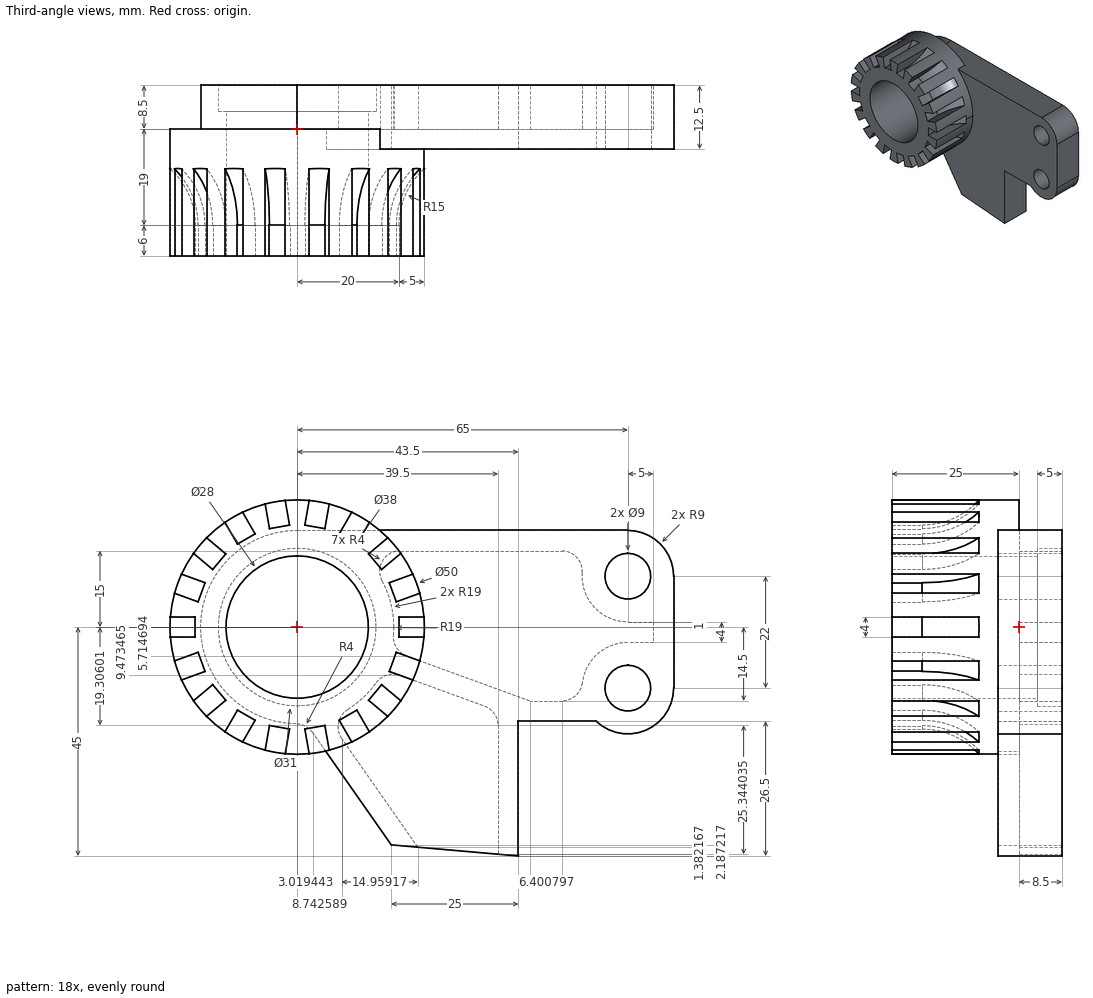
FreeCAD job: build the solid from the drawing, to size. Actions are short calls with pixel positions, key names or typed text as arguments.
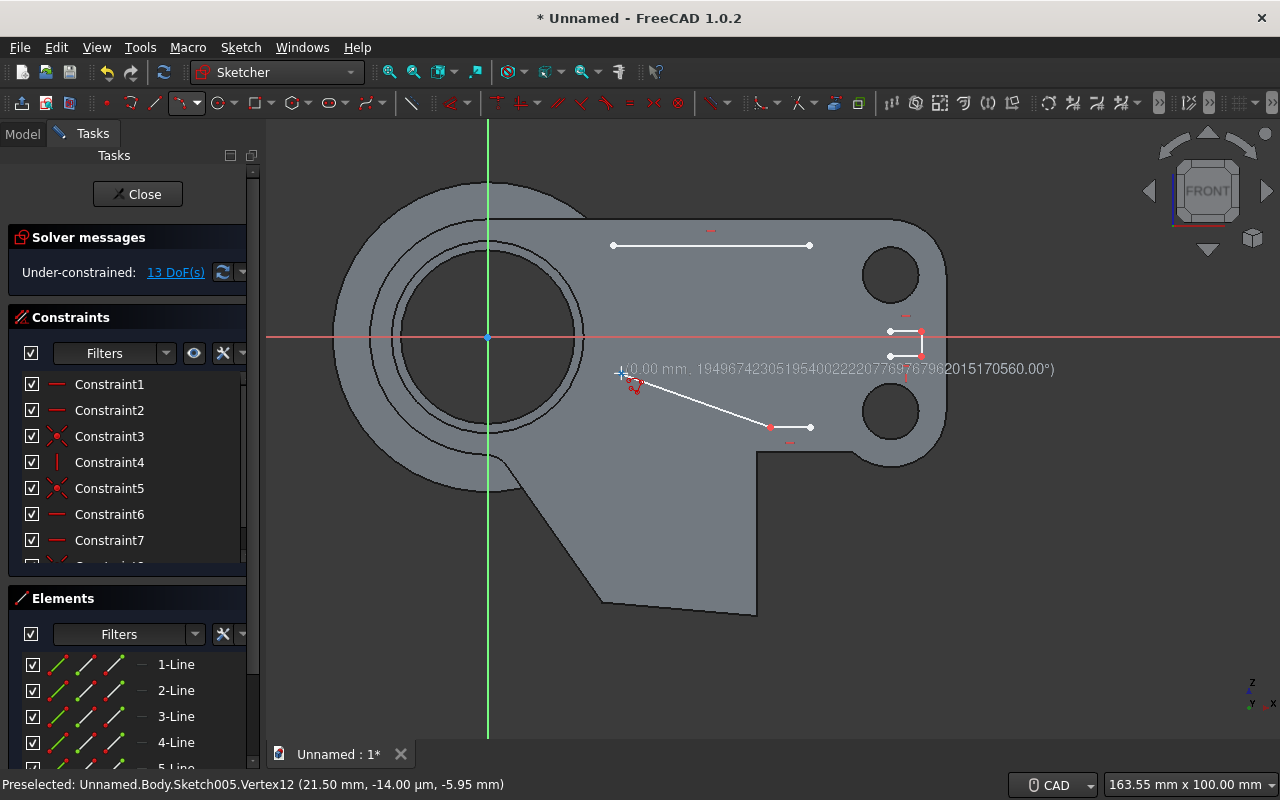
click(180, 104)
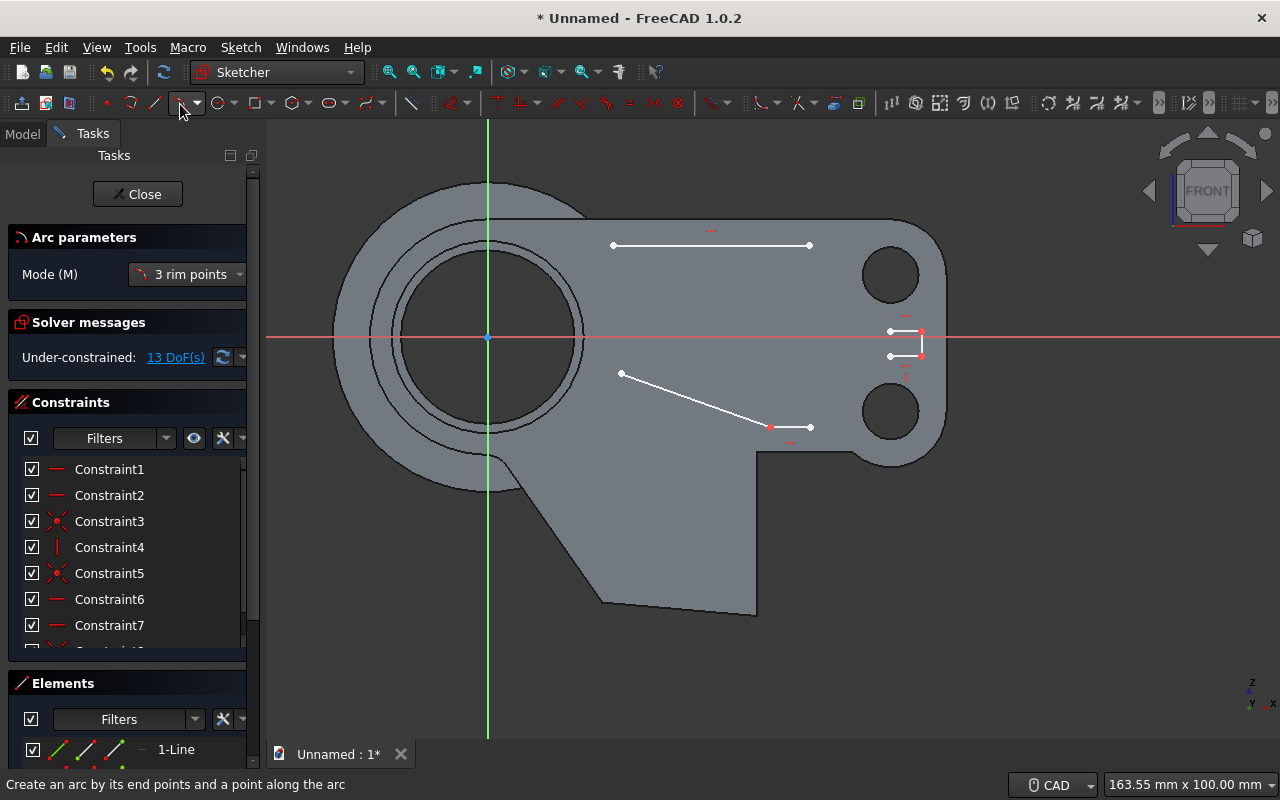
click(810, 246)
click(835, 271)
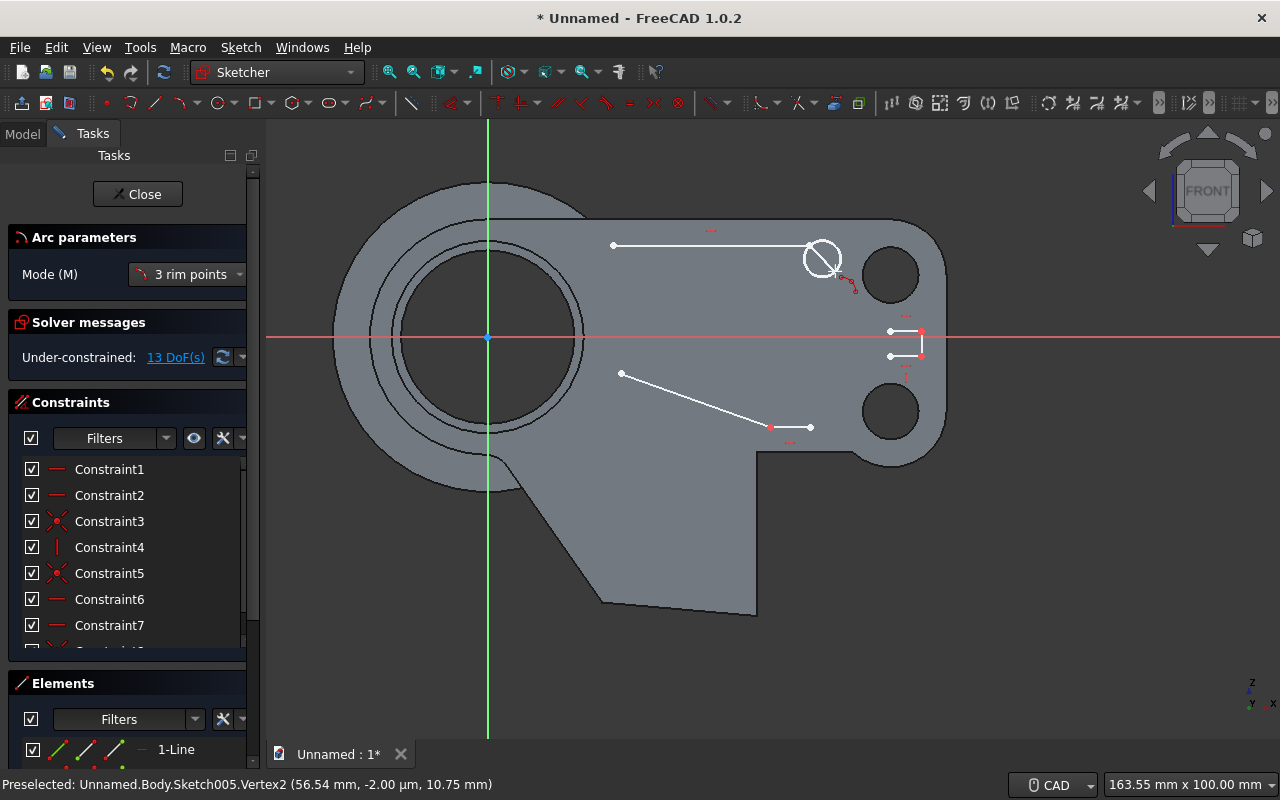
scroll(829, 252, up, 4)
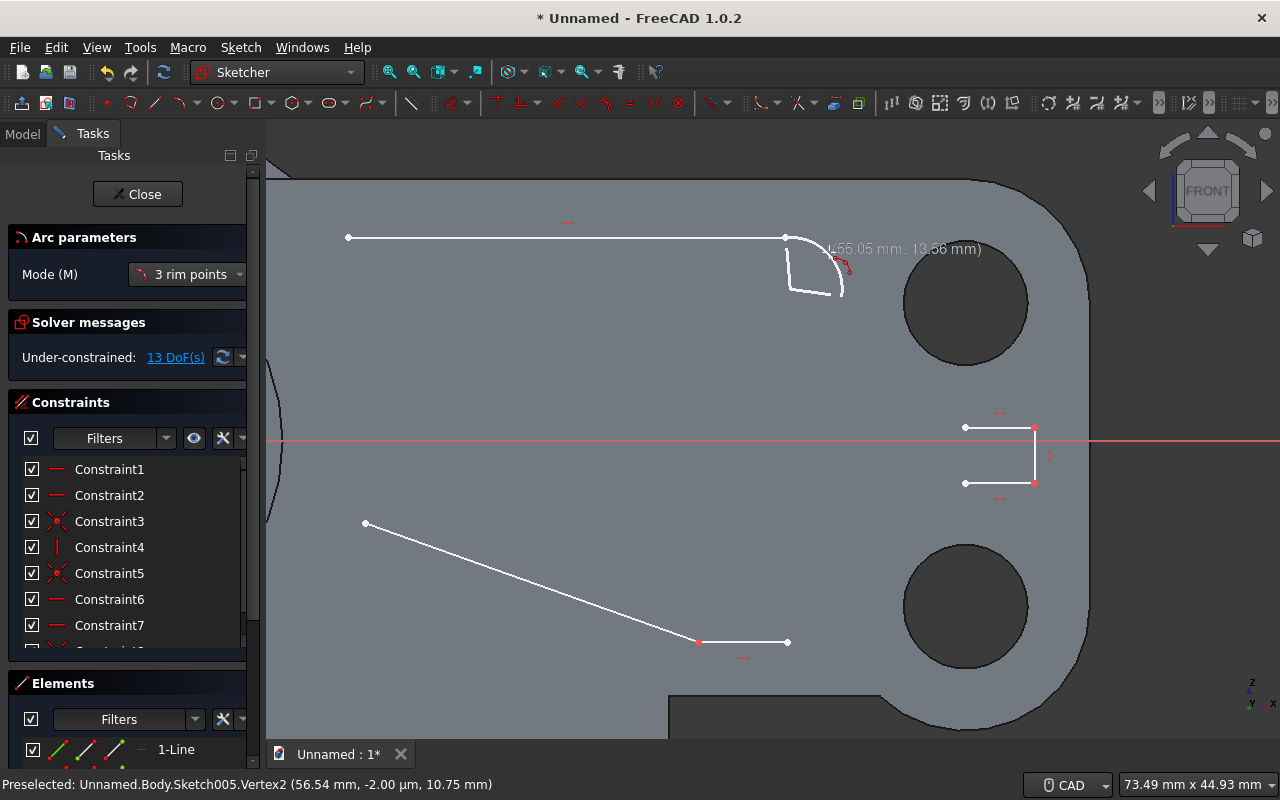
click(827, 252)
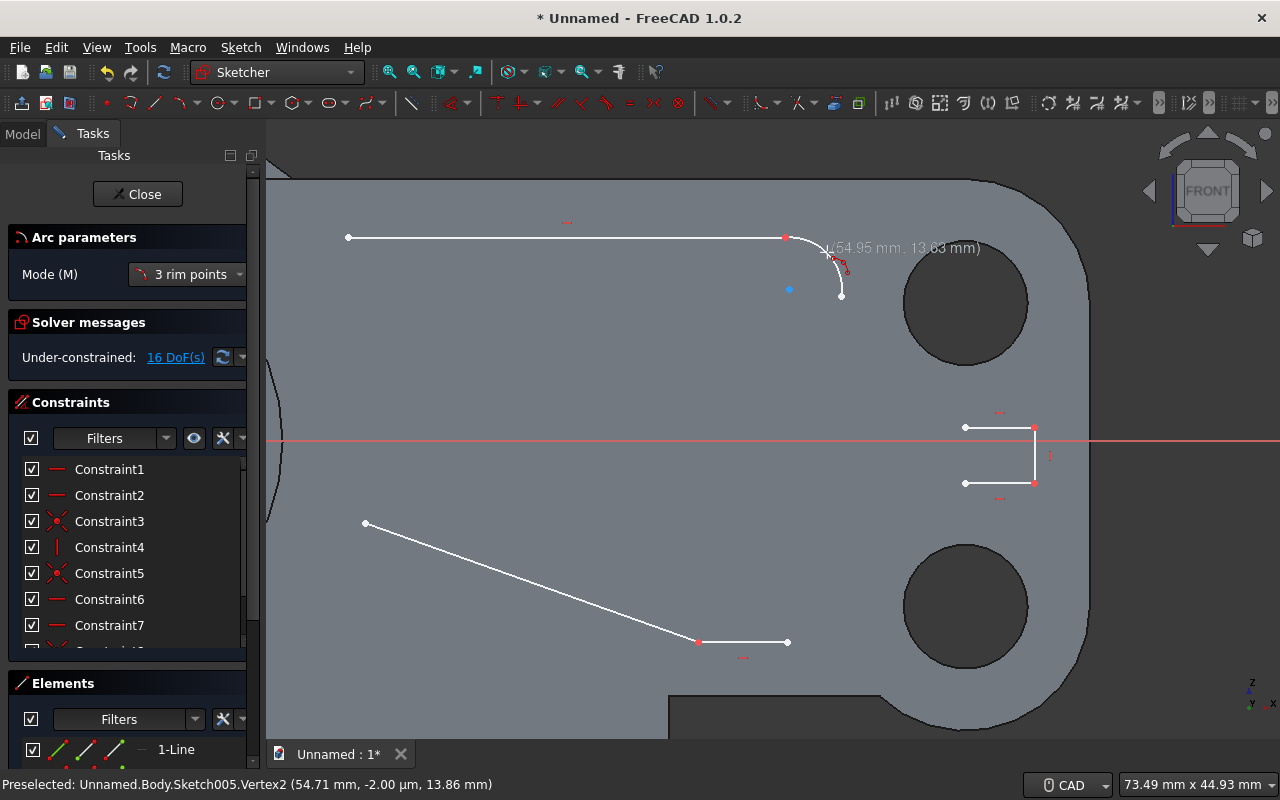
click(842, 296)
click(966, 428)
click(875, 388)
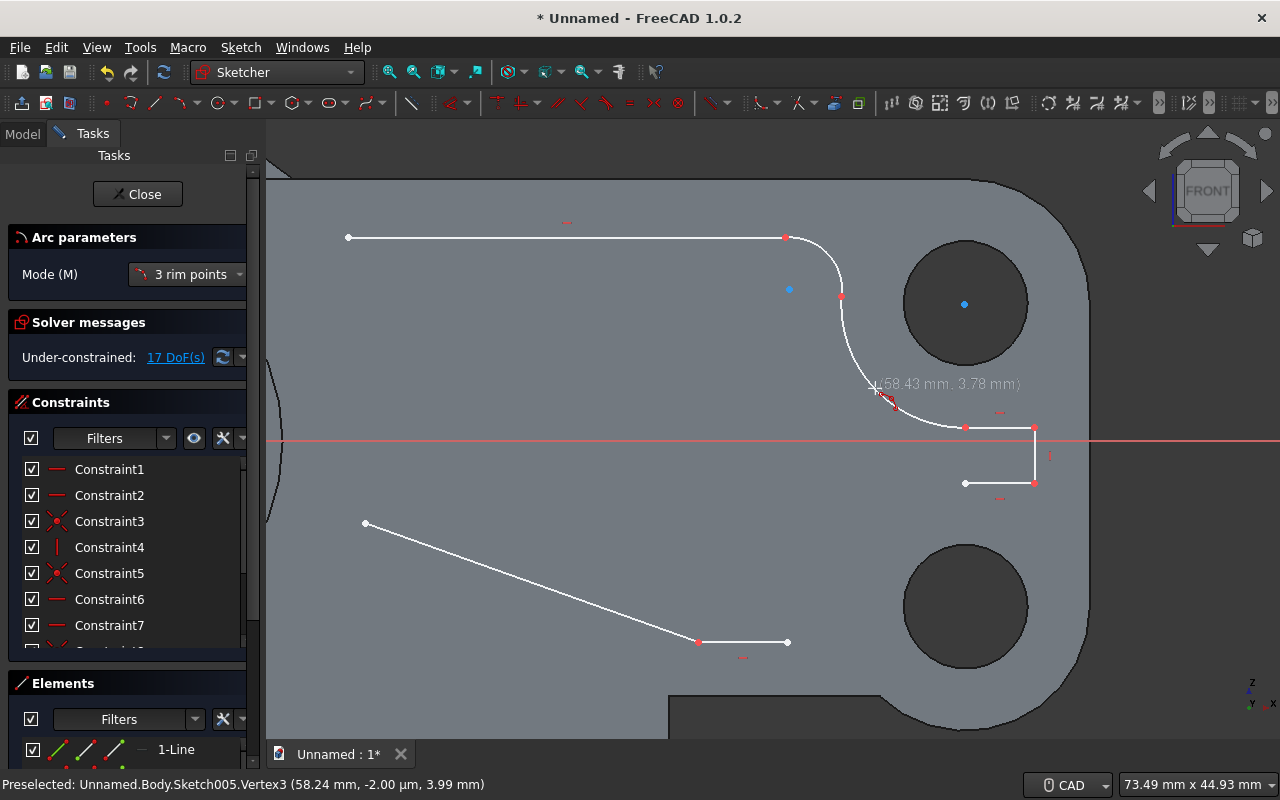
click(966, 483)
click(842, 592)
click(883, 514)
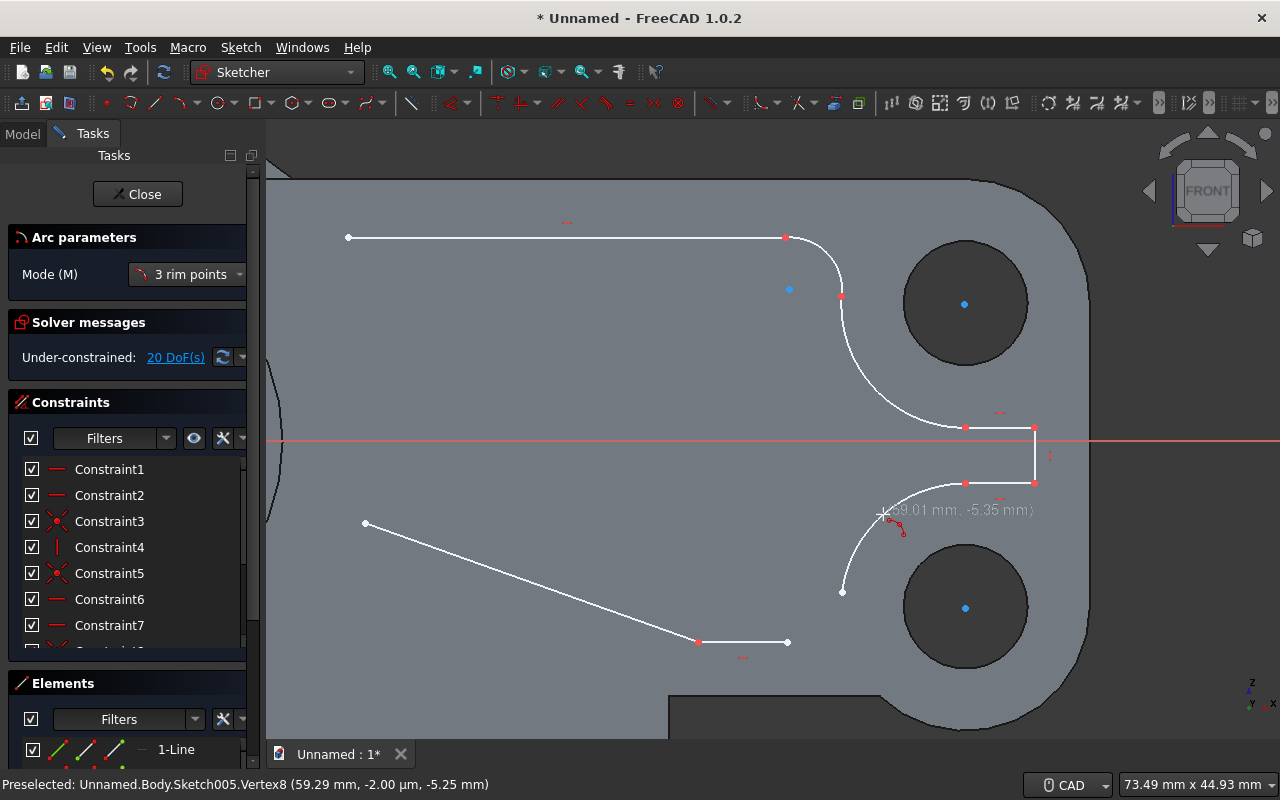
click(842, 593)
click(787, 642)
click(824, 627)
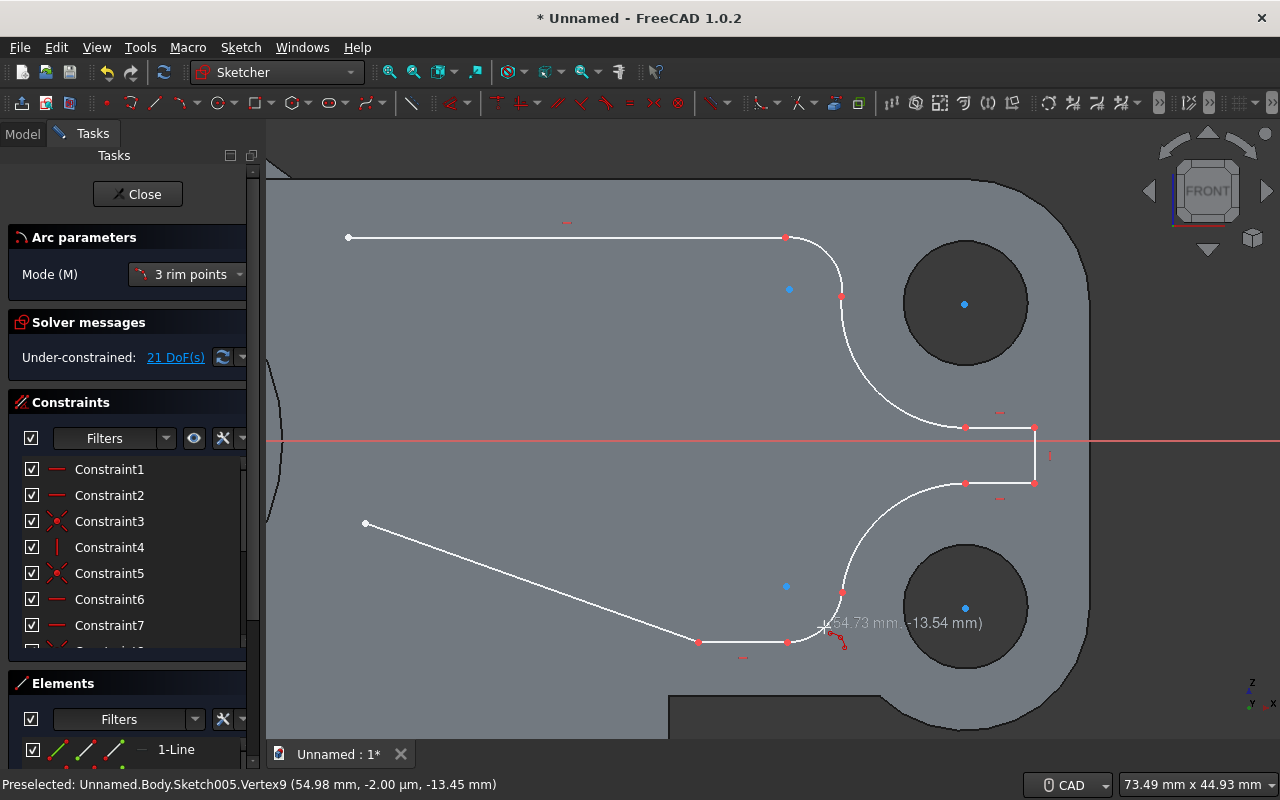
click(365, 523)
click(330, 463)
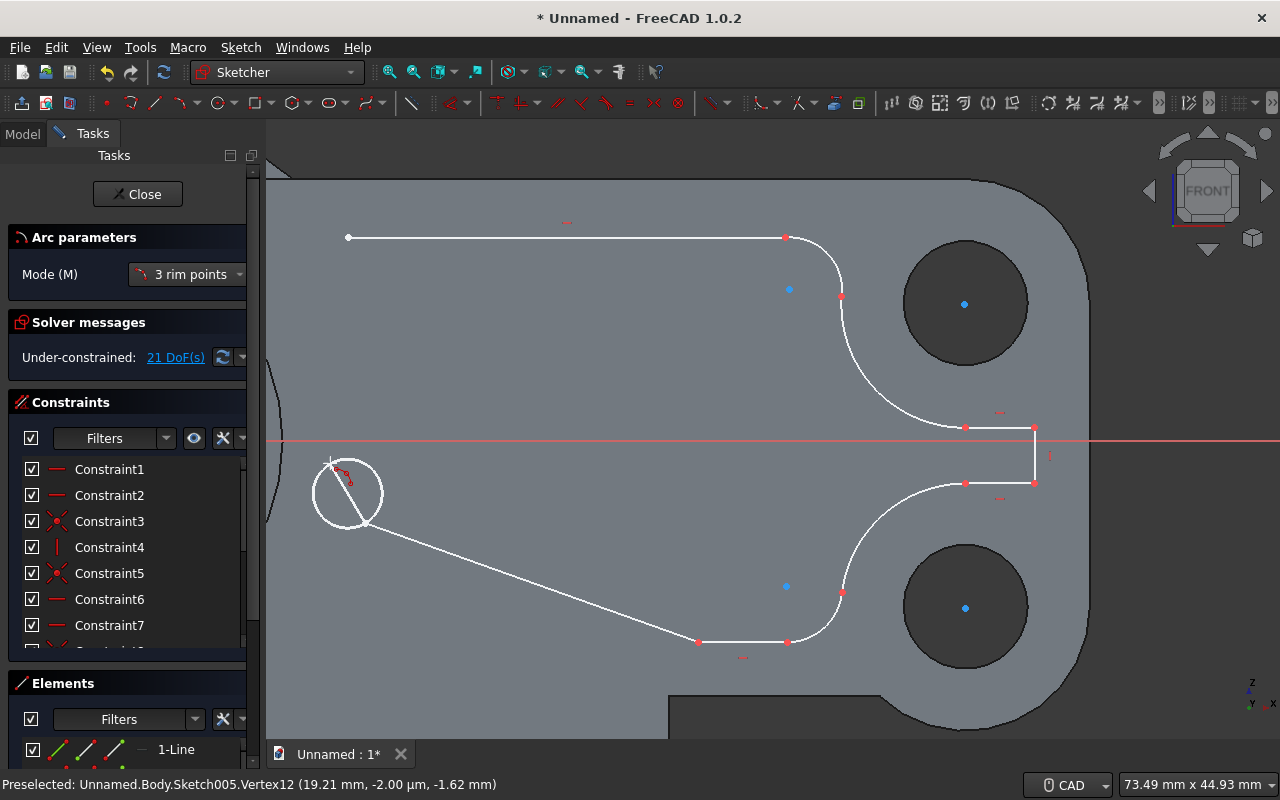
scroll(338, 498, up, 2)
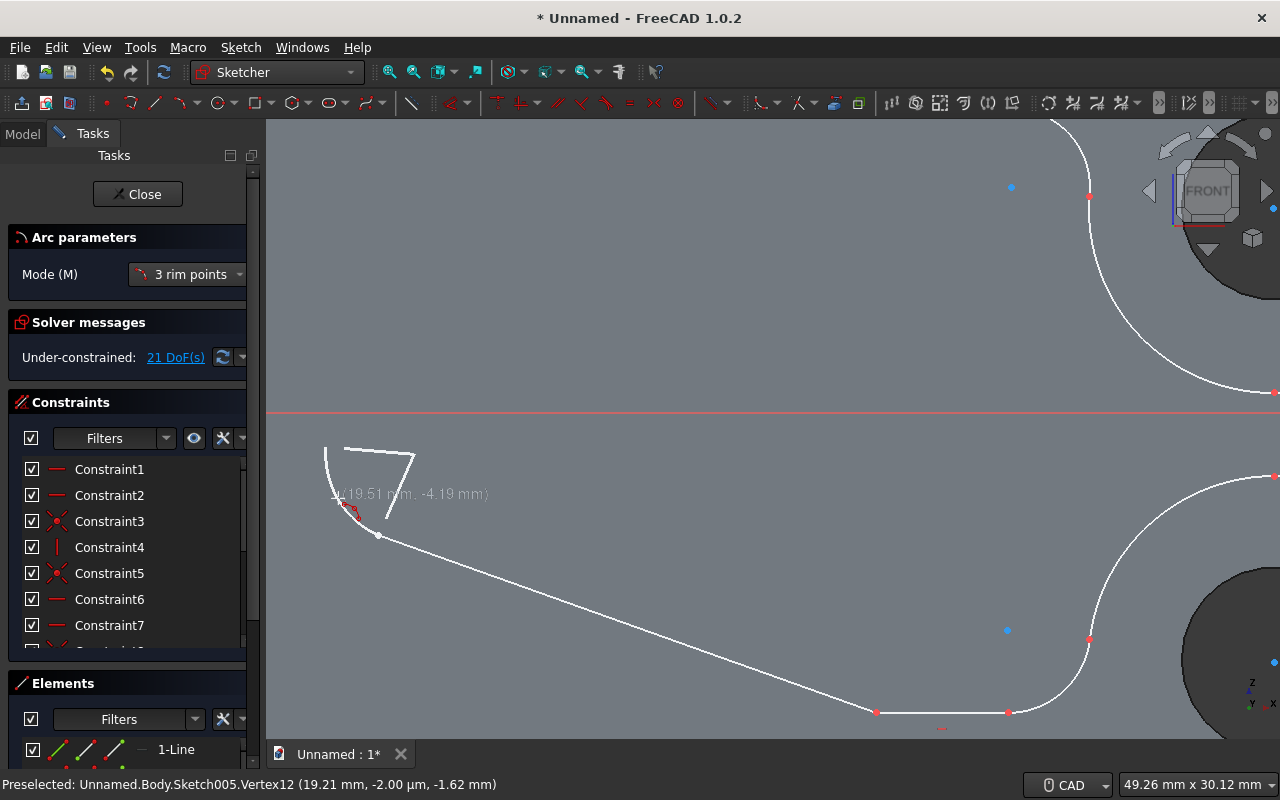
click(339, 497)